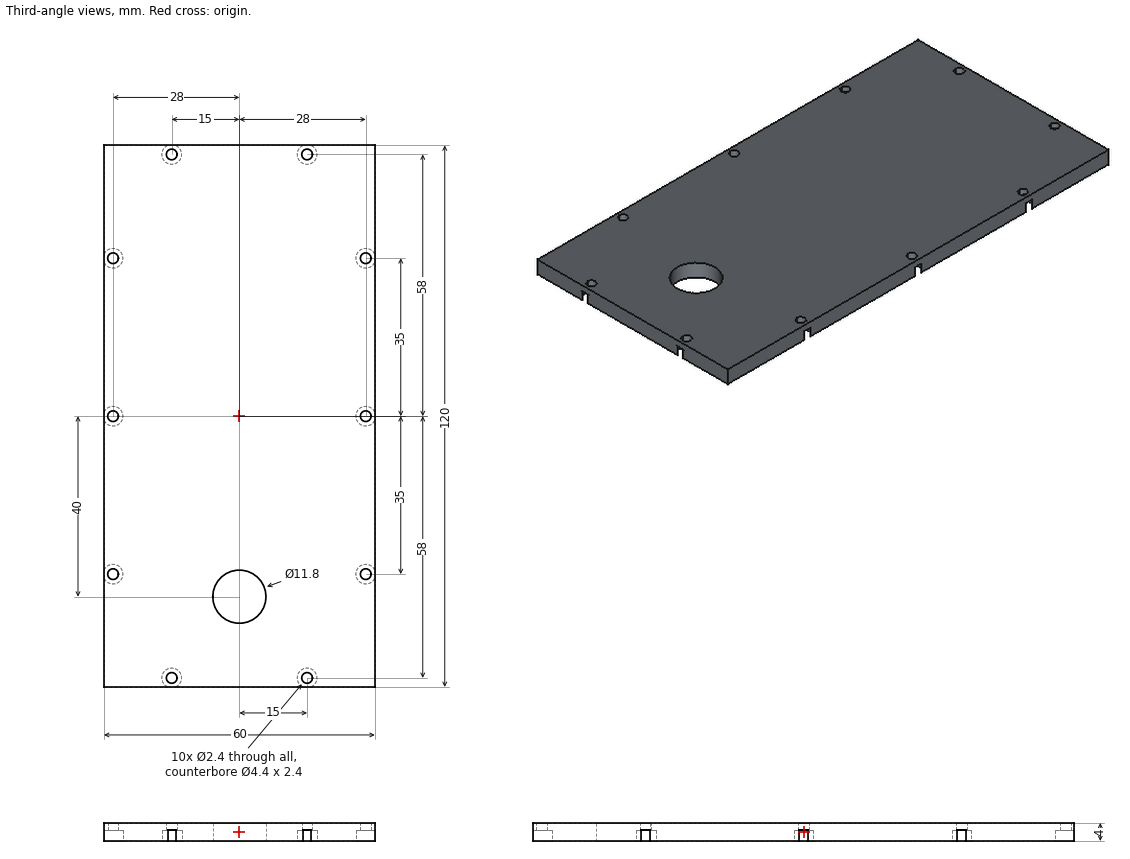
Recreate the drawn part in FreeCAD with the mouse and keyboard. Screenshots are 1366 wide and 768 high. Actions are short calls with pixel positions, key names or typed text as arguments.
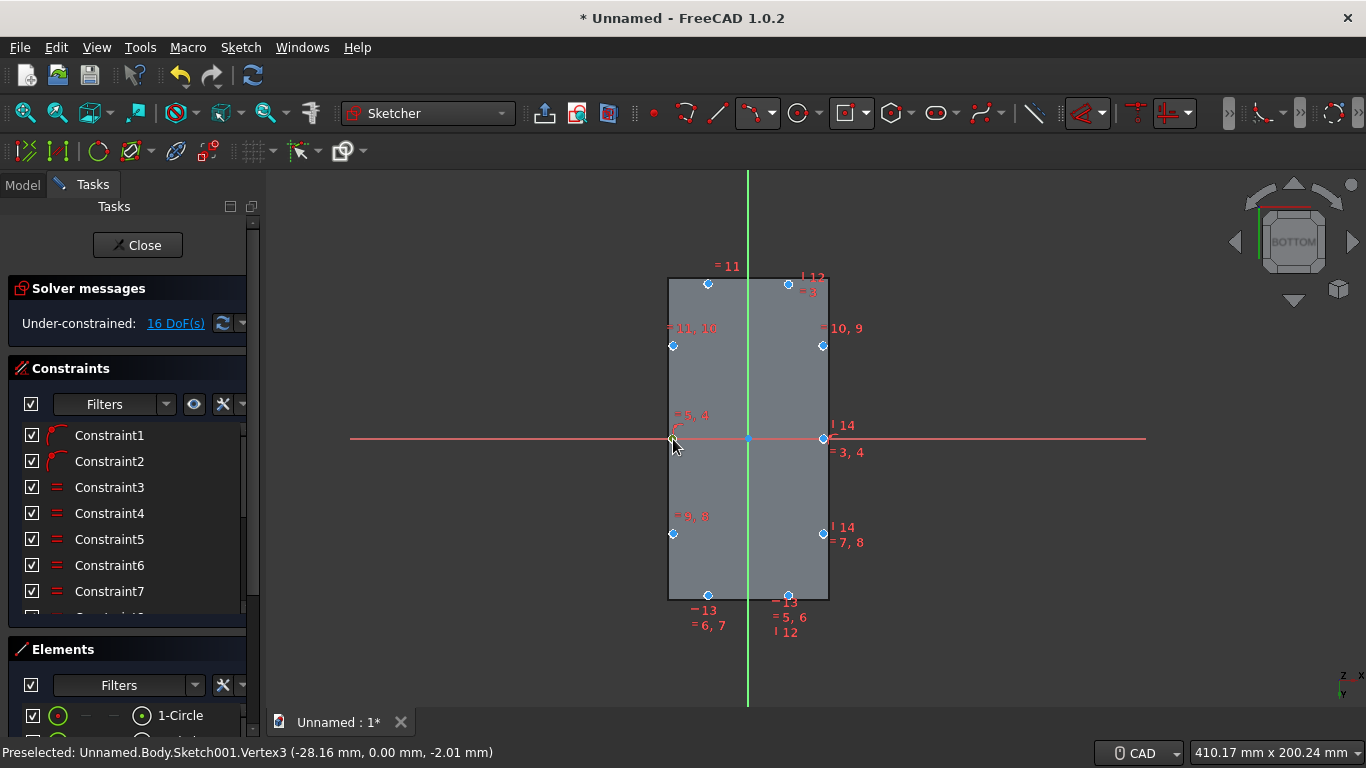
click(673, 534)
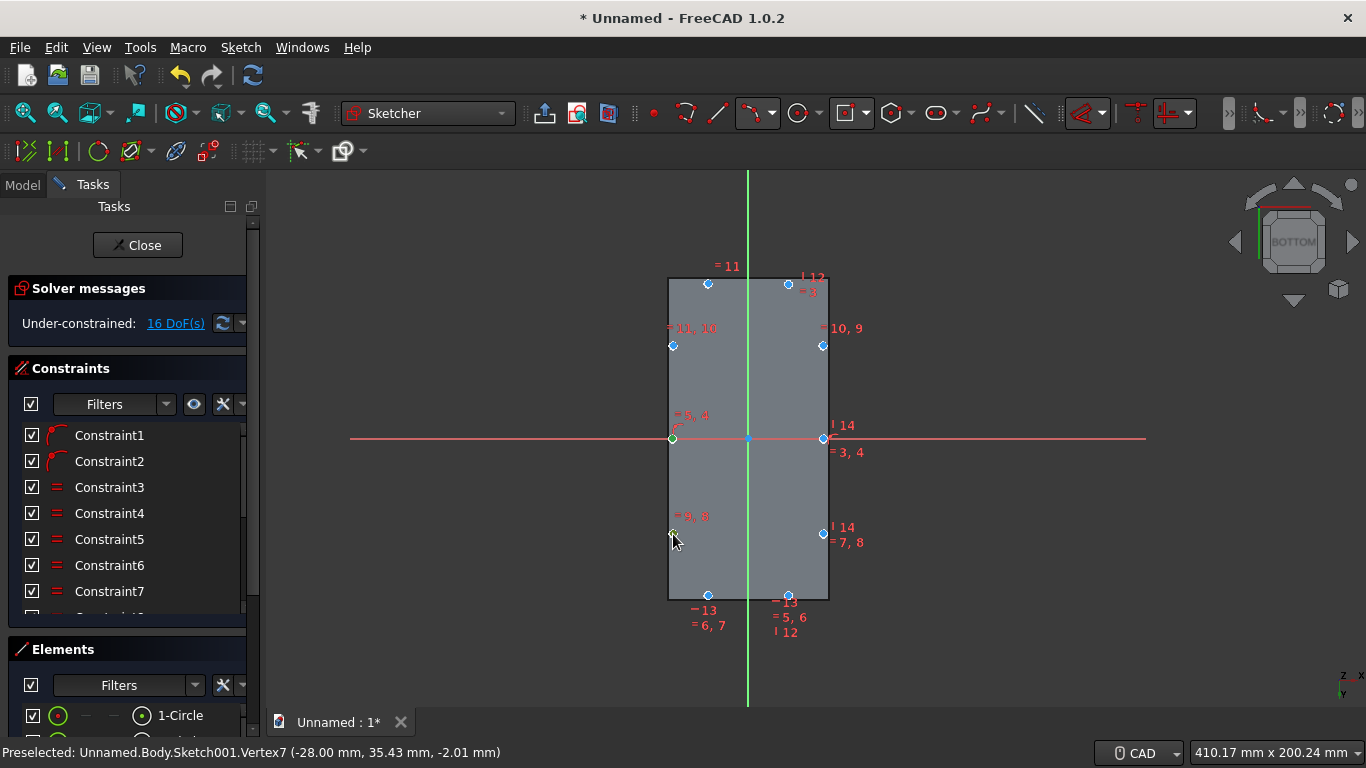
click(1190, 114)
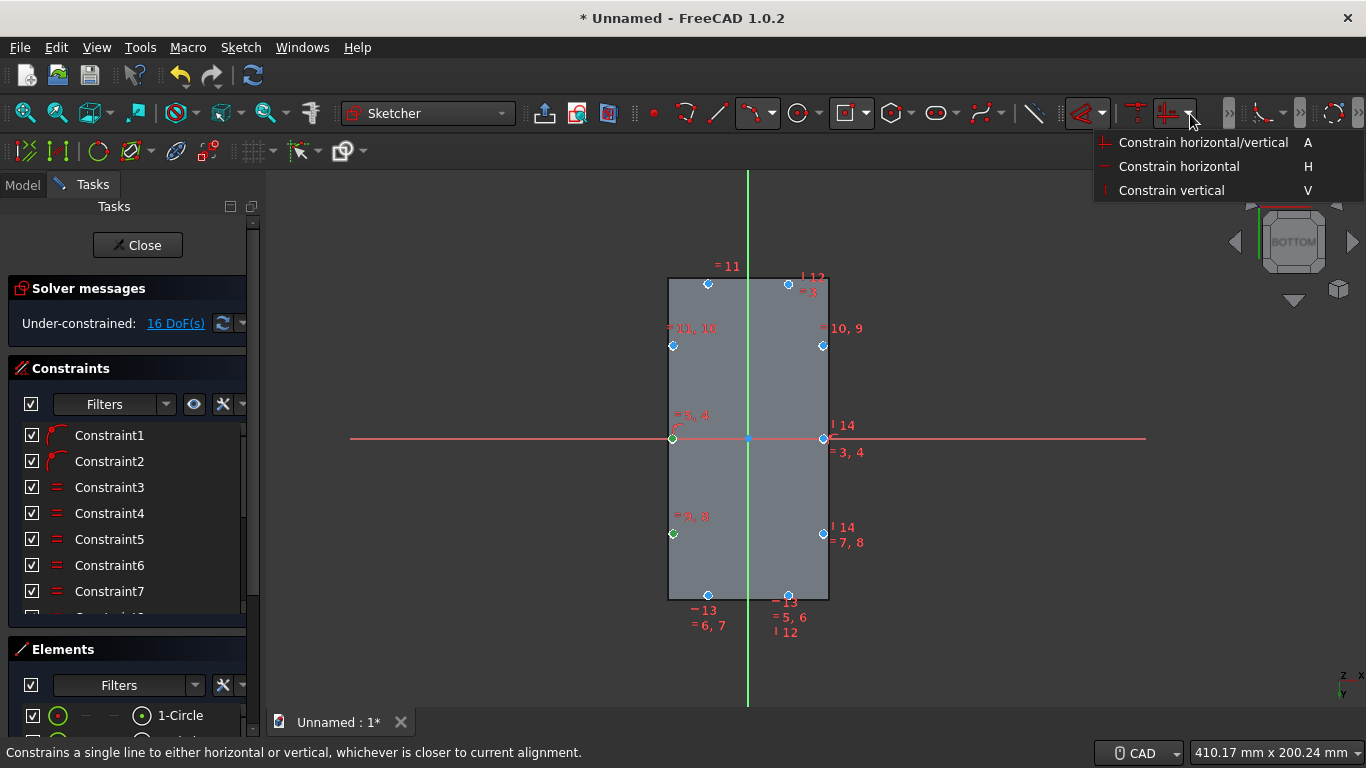
click(1229, 190)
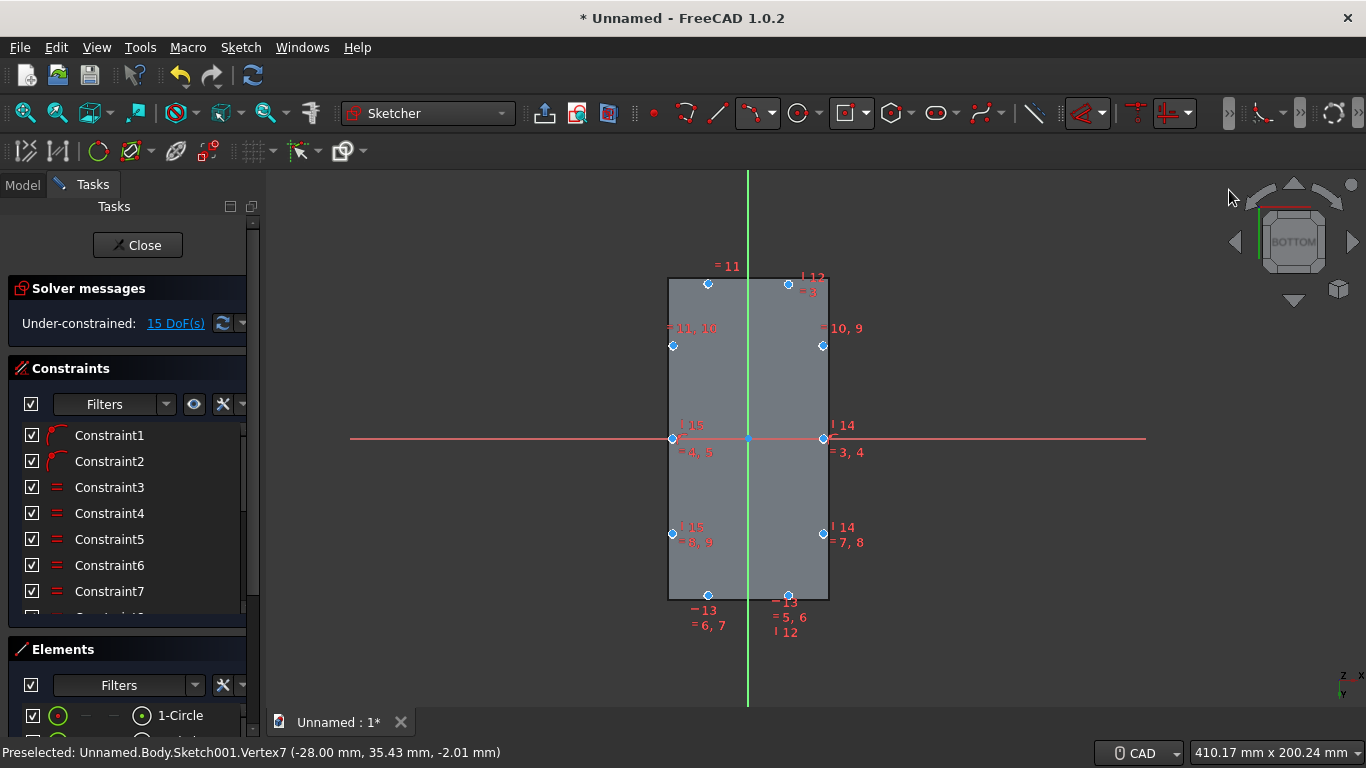
click(824, 534)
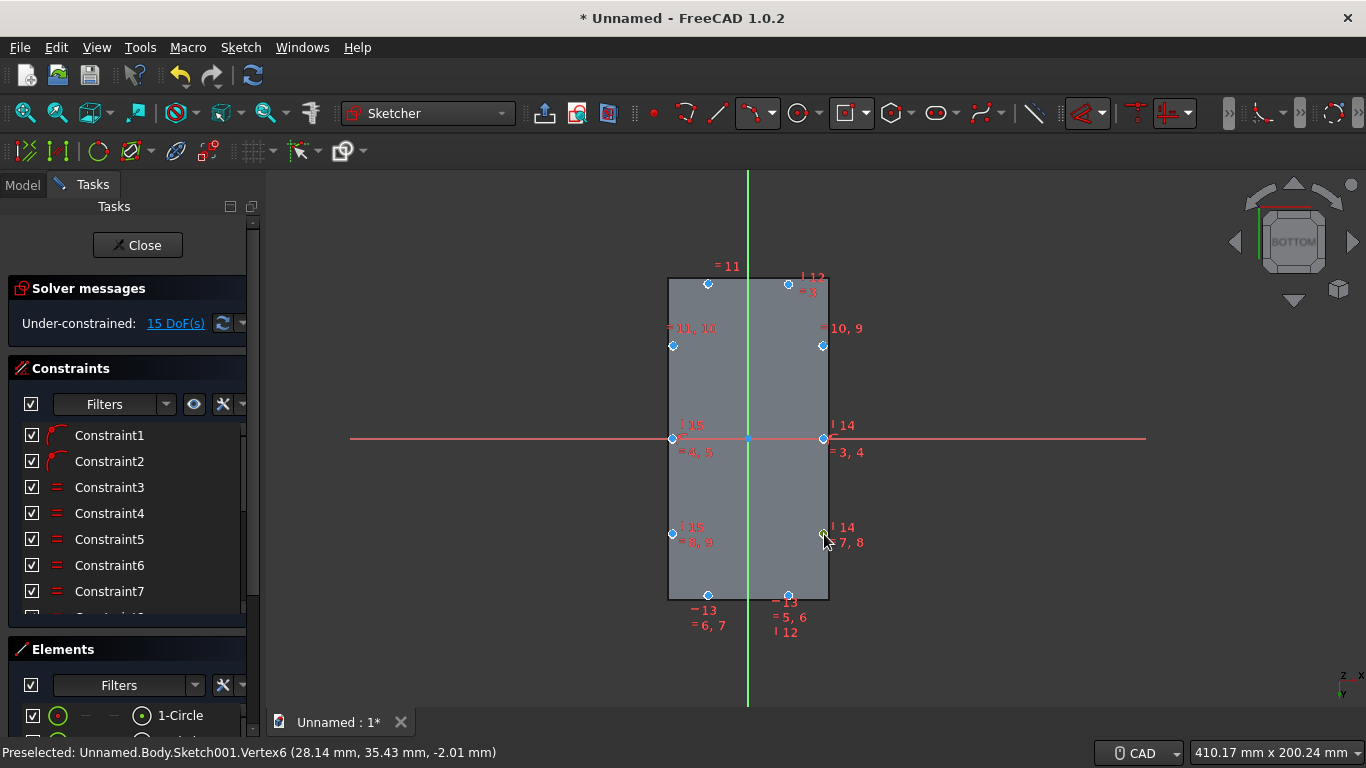
click(673, 534)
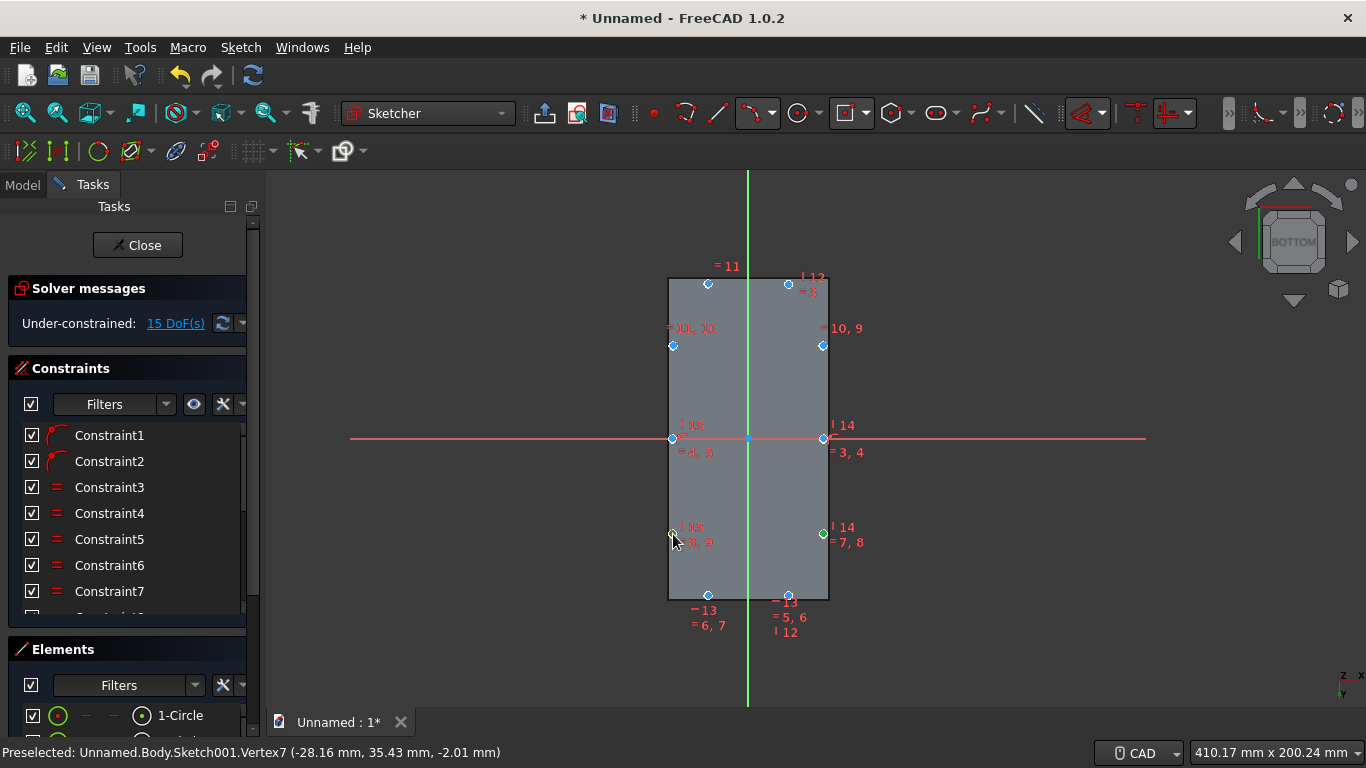
click(1190, 114)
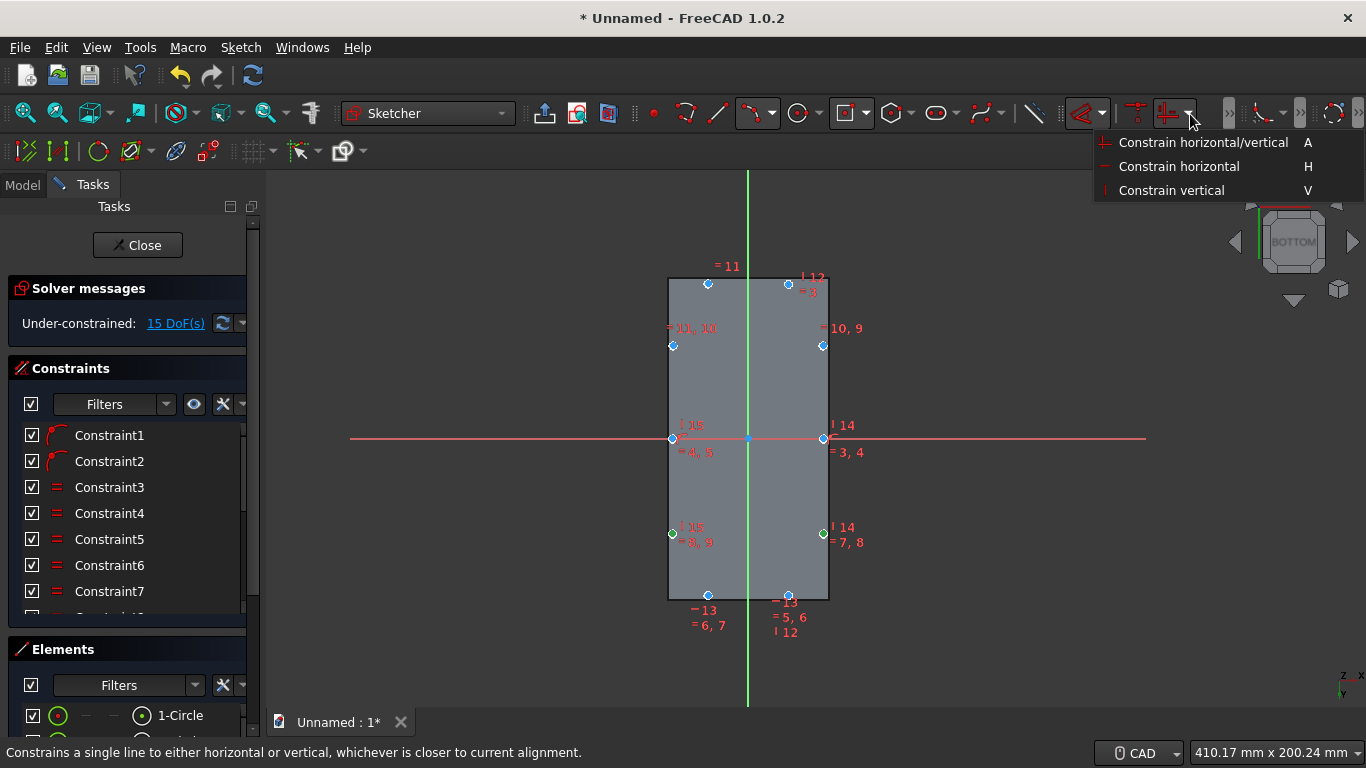
click(1229, 166)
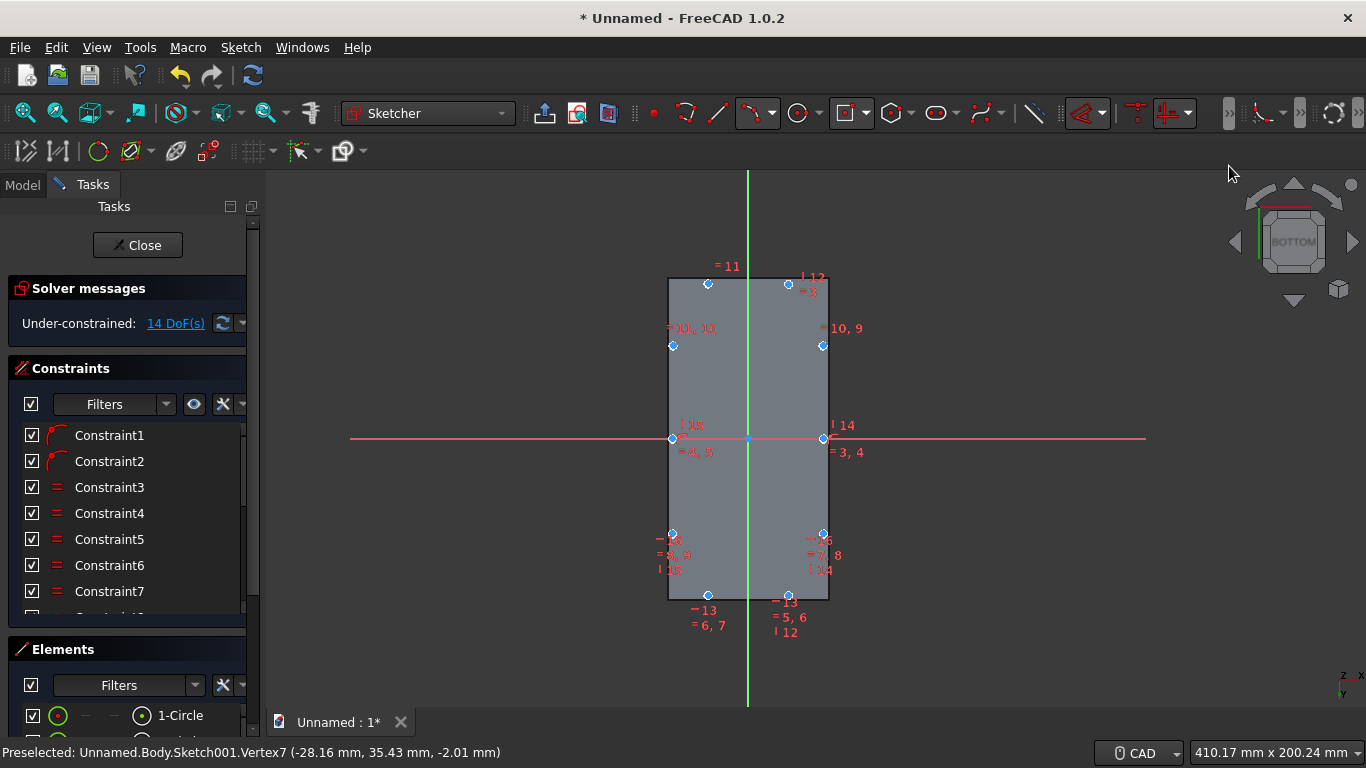
click(824, 439)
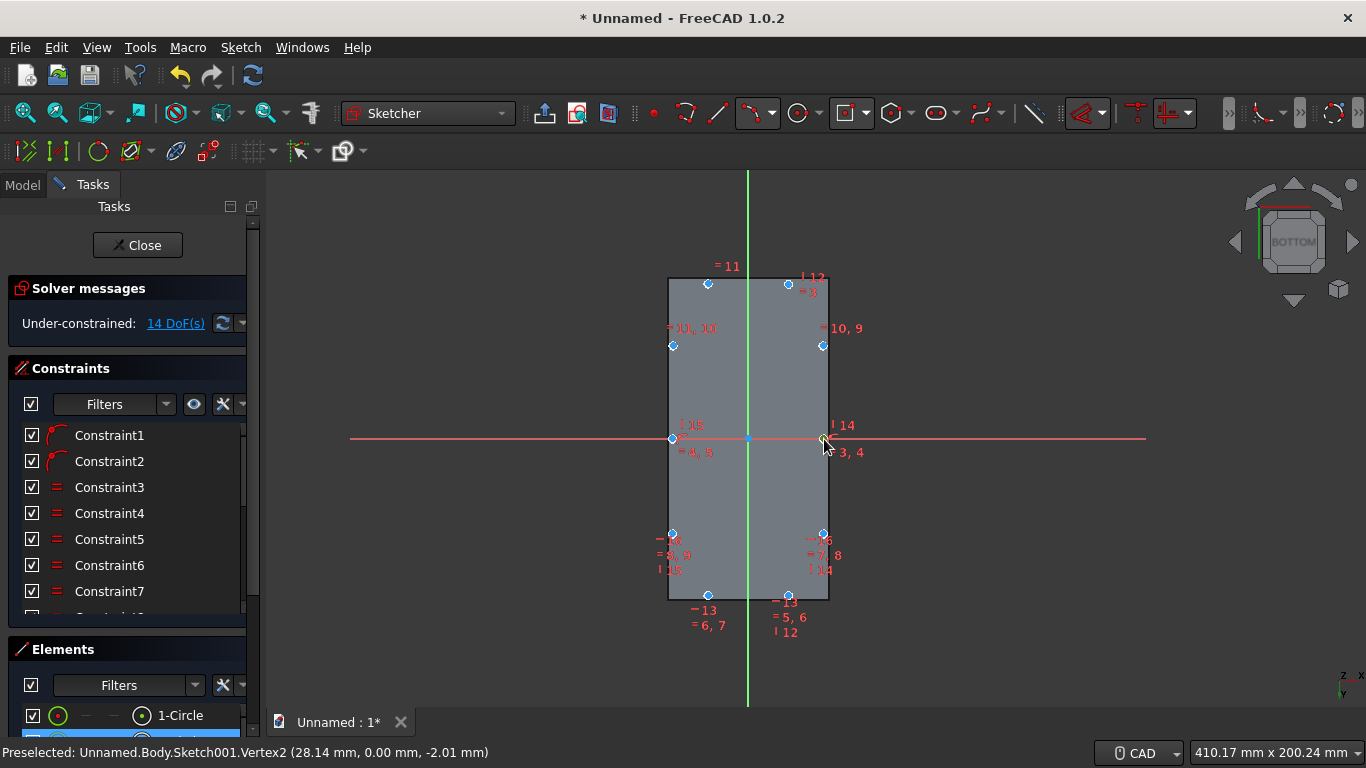
click(823, 346)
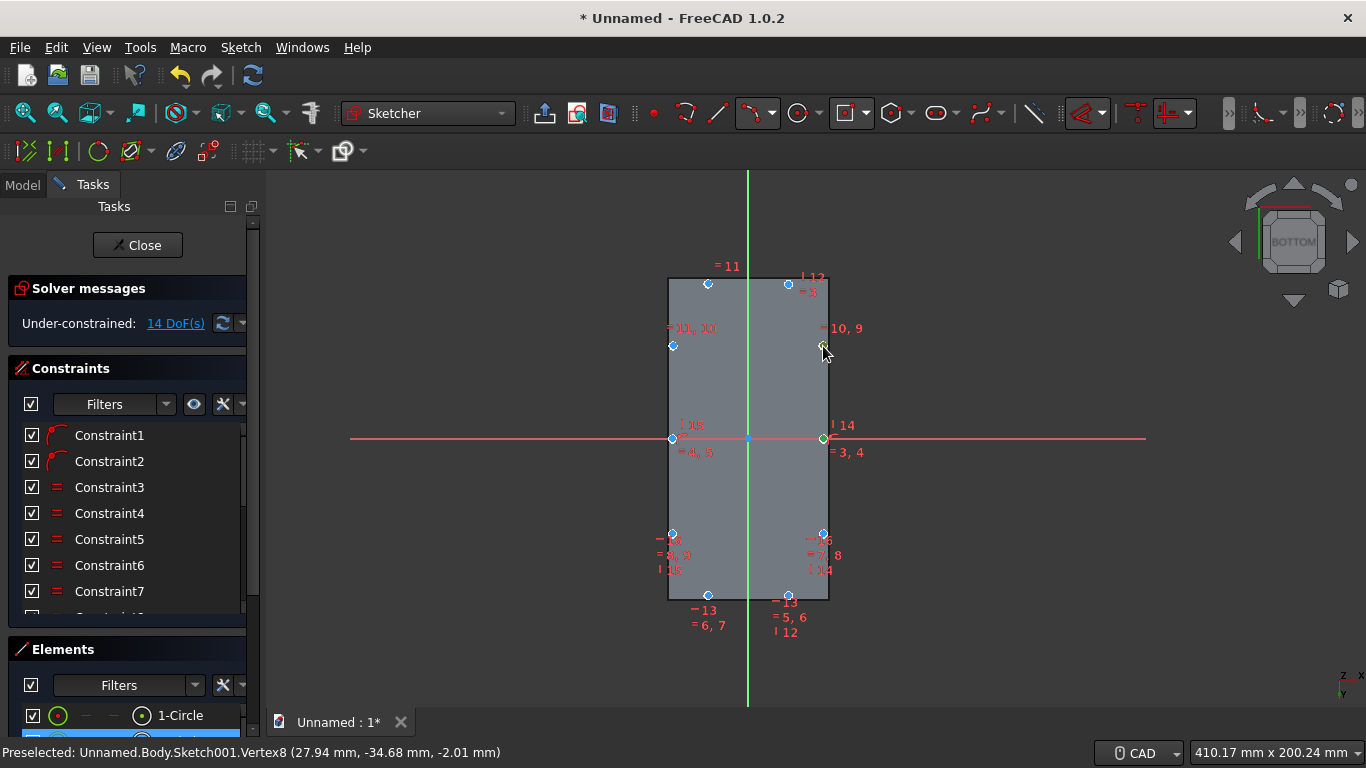
key(v)